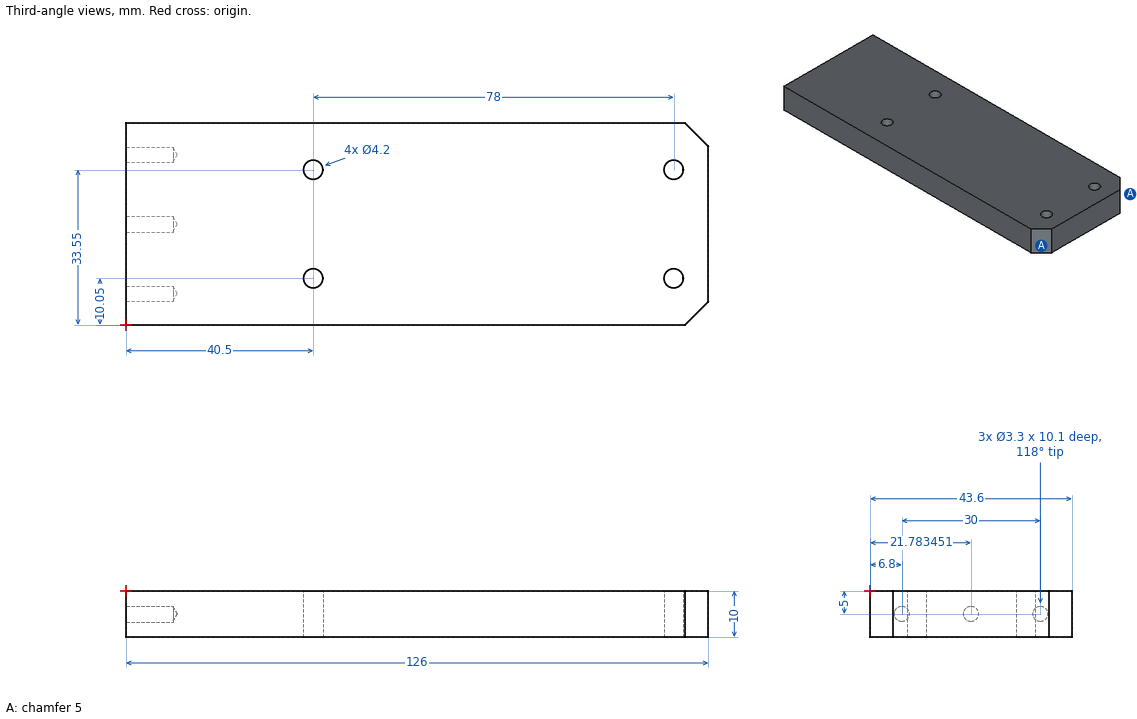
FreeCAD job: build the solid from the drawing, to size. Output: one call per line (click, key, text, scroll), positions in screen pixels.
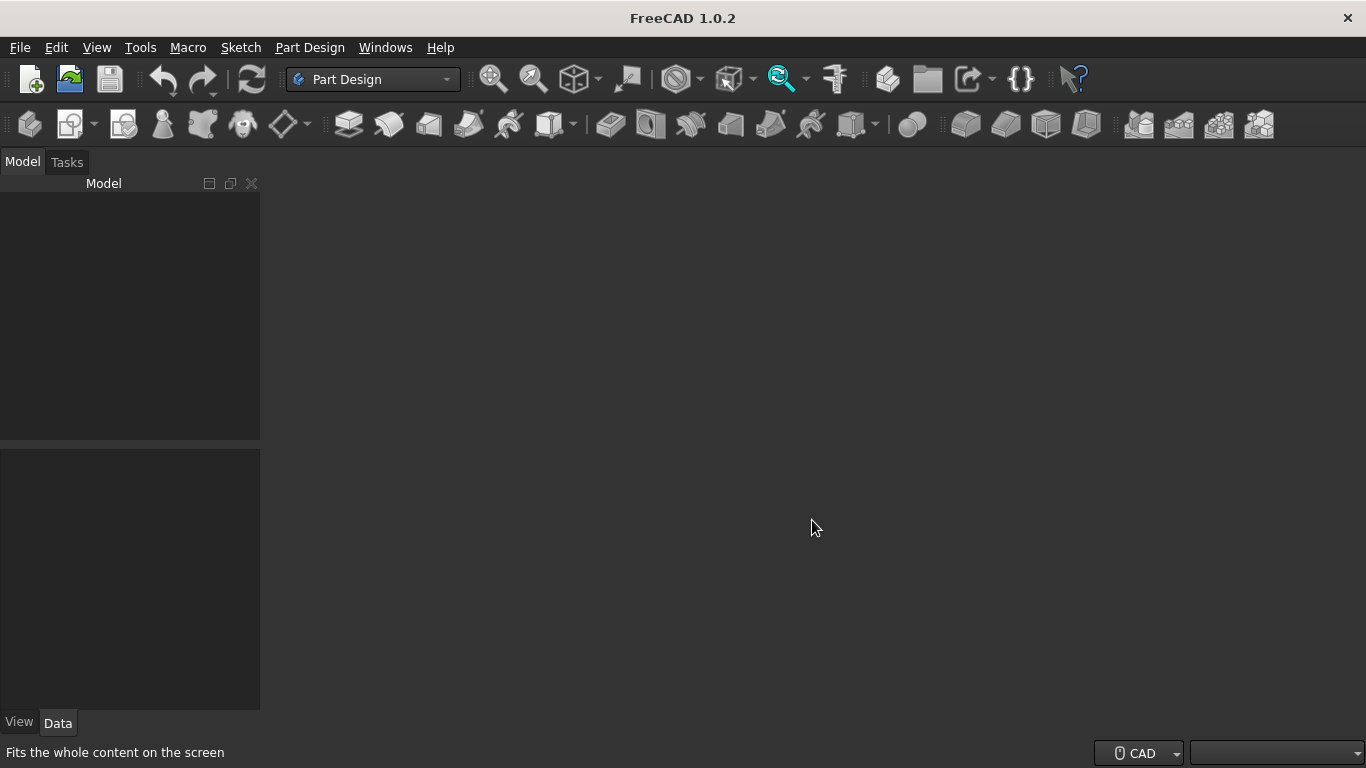
click(30, 80)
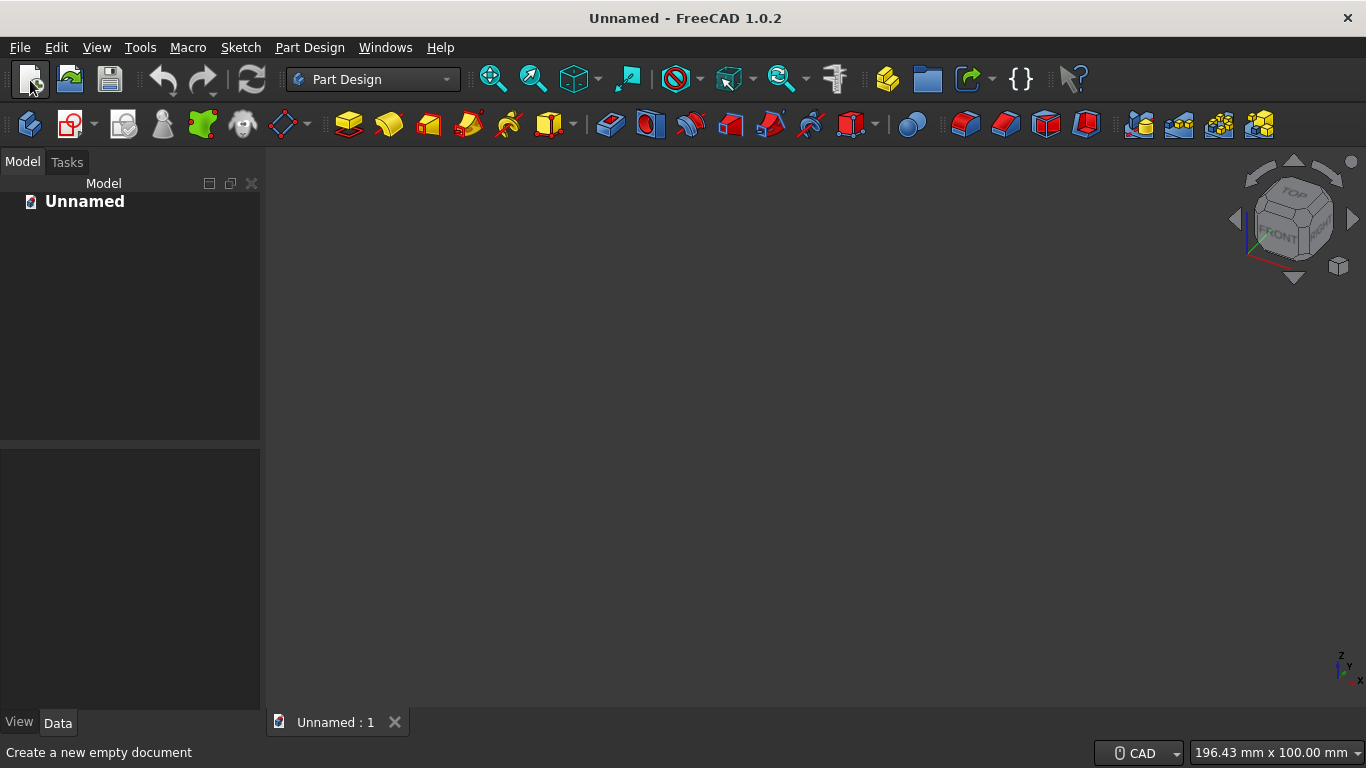
click(70, 124)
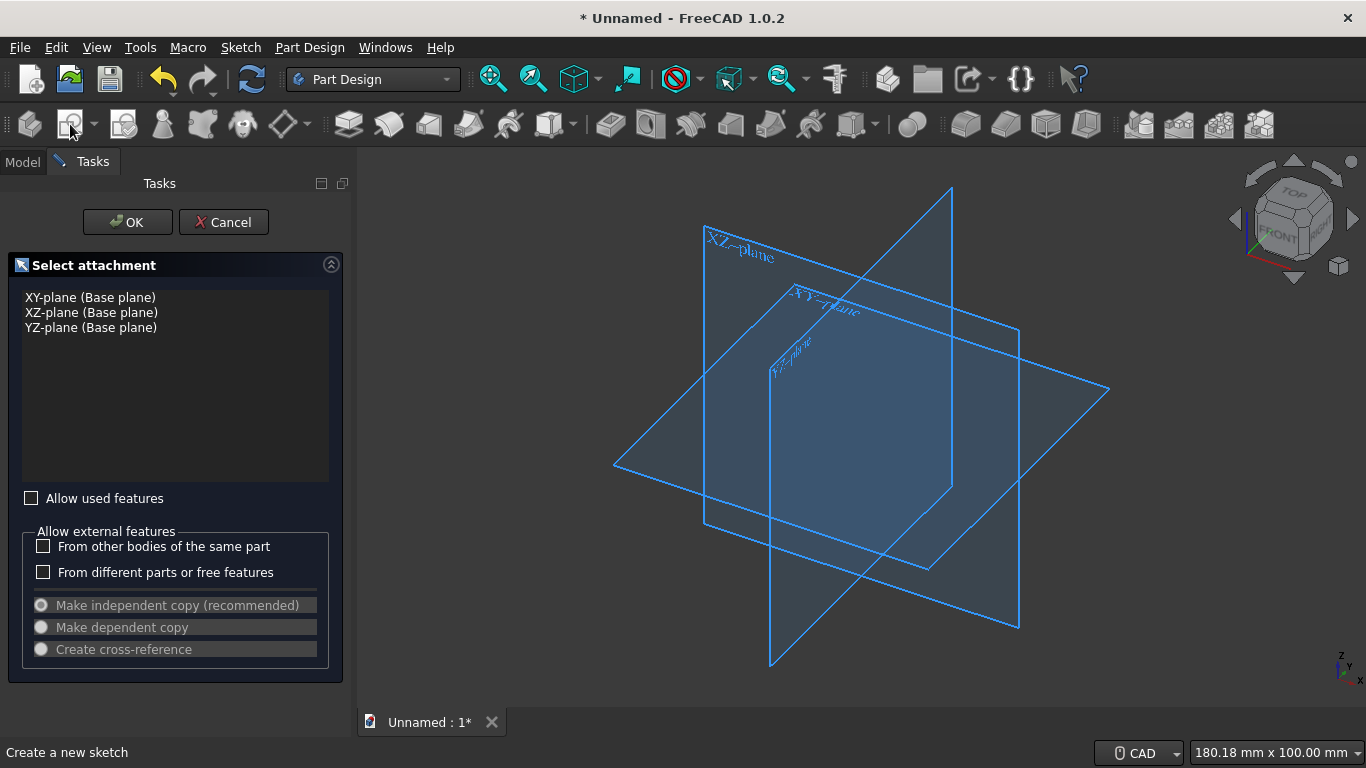
click(82, 312)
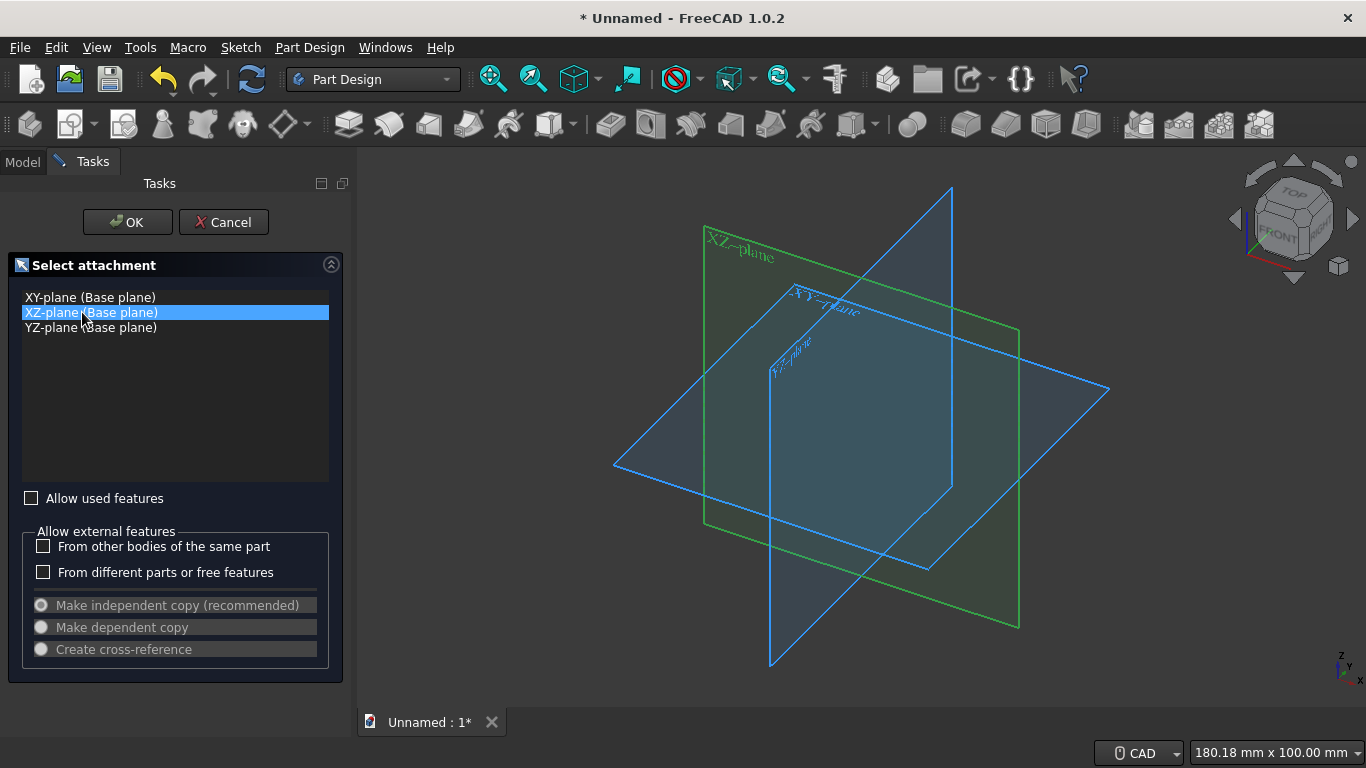
click(128, 222)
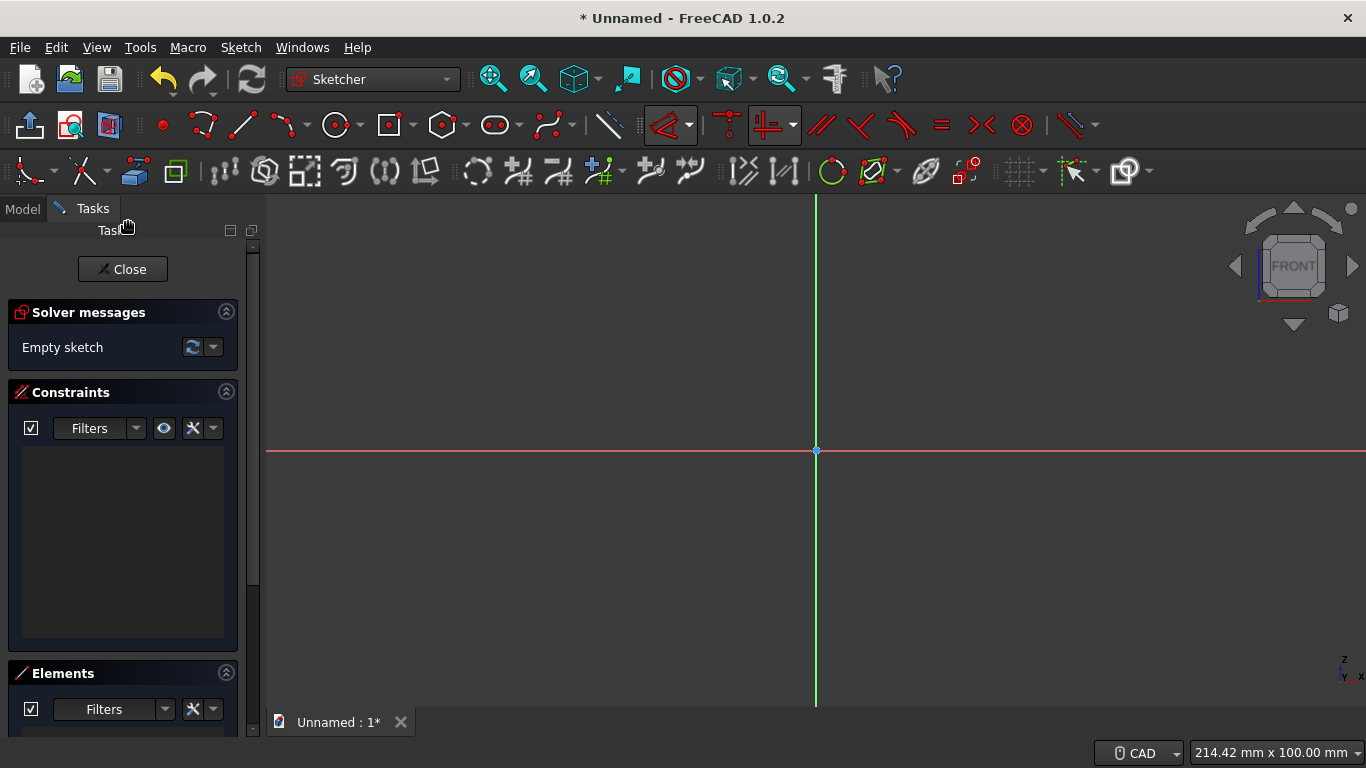
scroll(294, 398, down, 2)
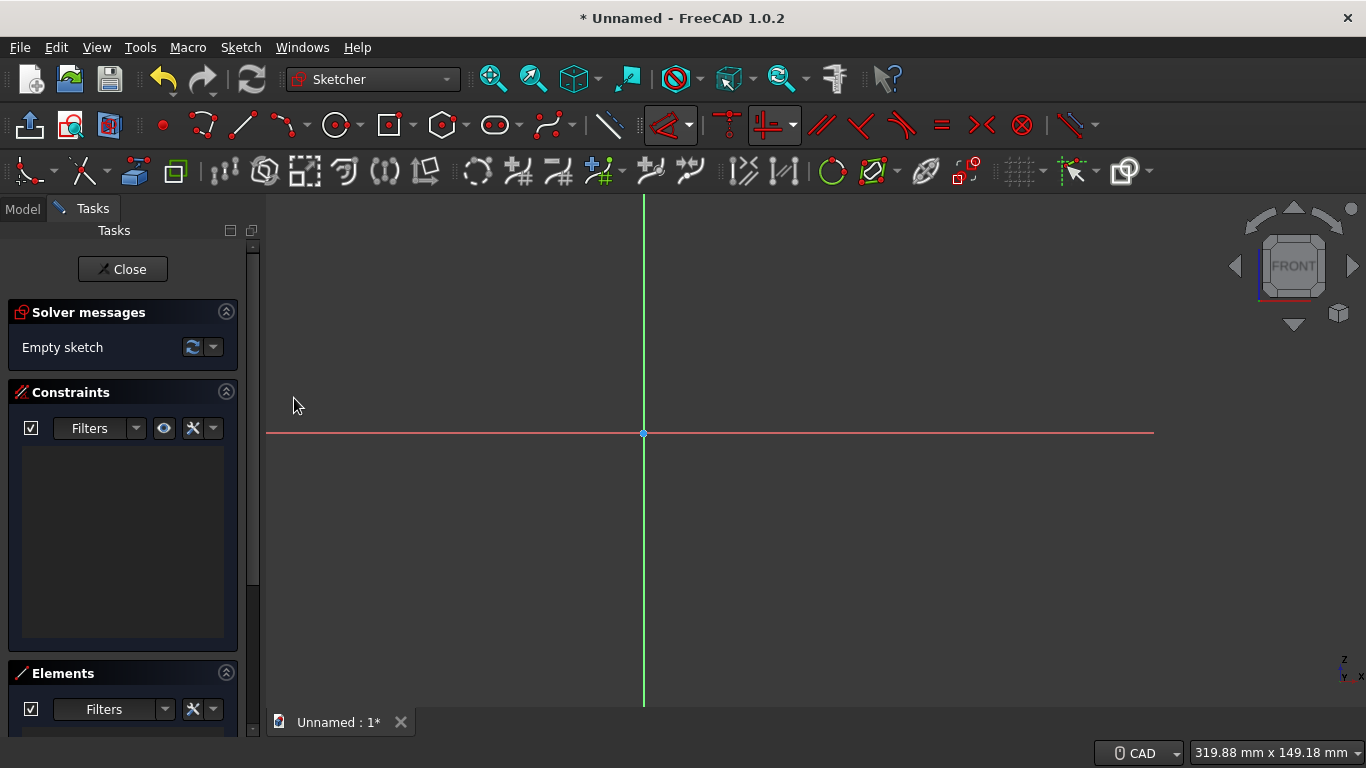
scroll(1090, 451, up, 2)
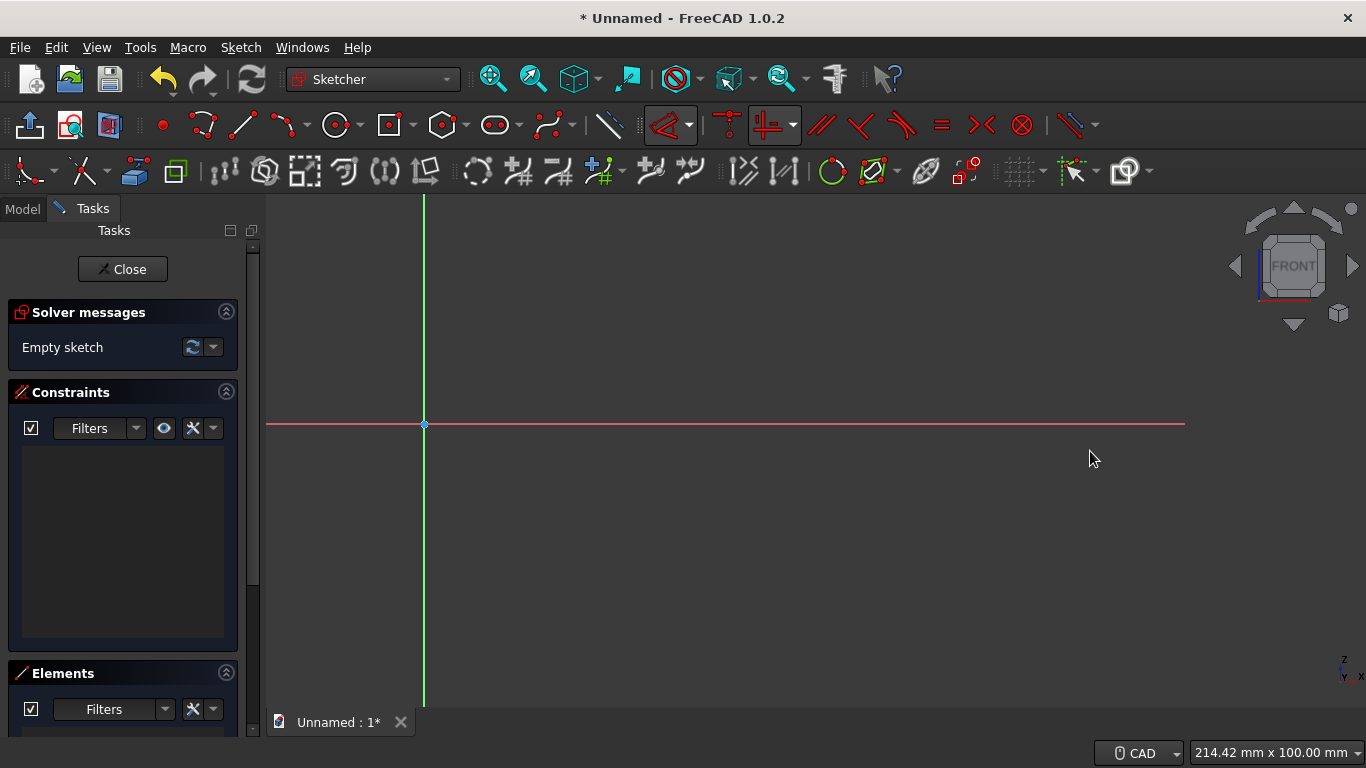
key(g)
key(r)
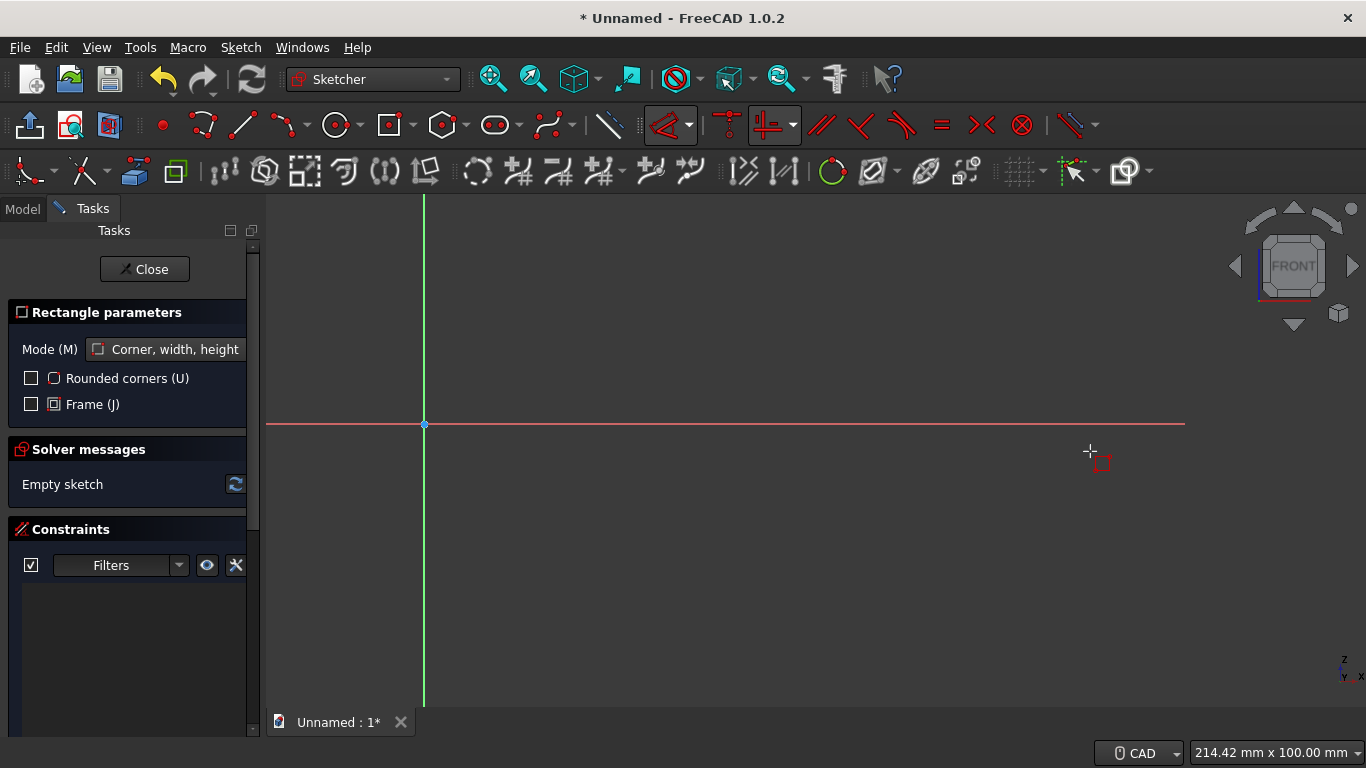
click(424, 424)
move(1071, 476)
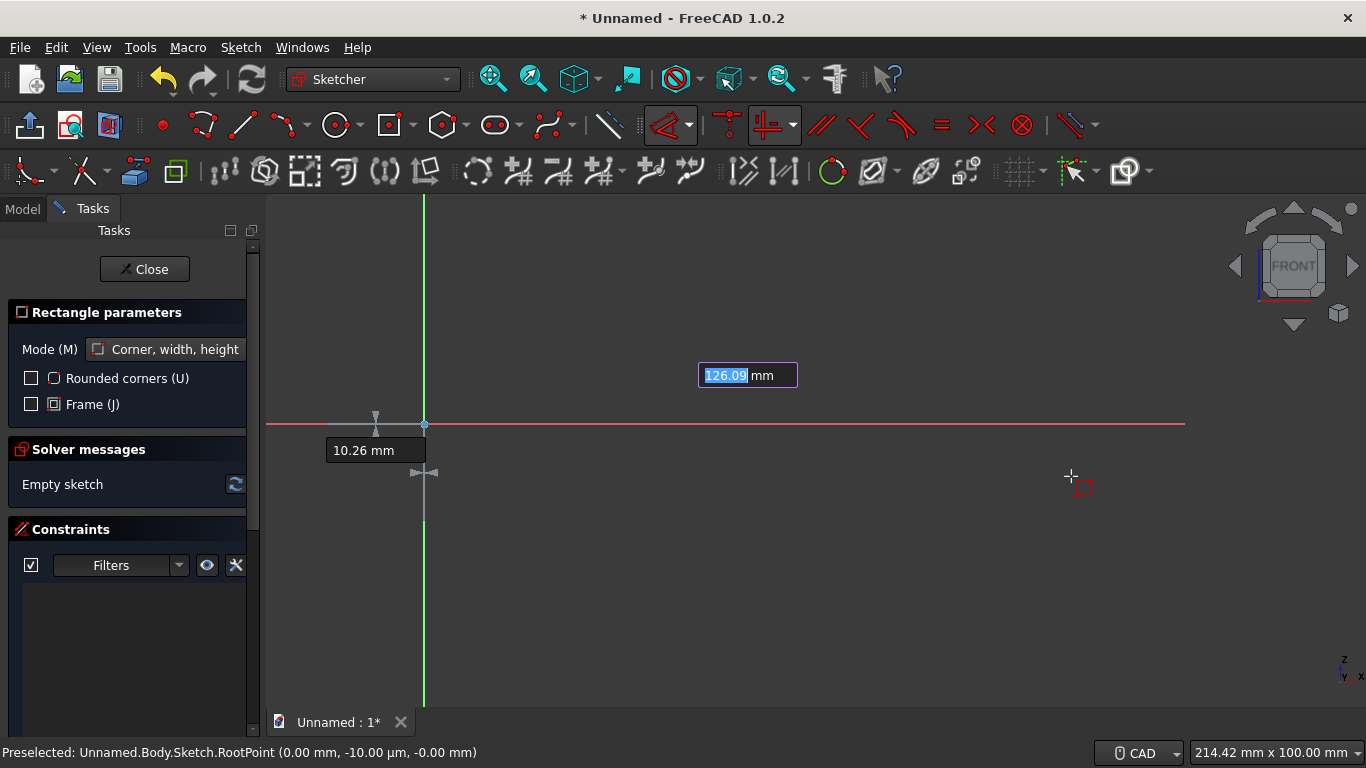
text(126)
key(Tab)
text(10)
key(Return)
key(Escape)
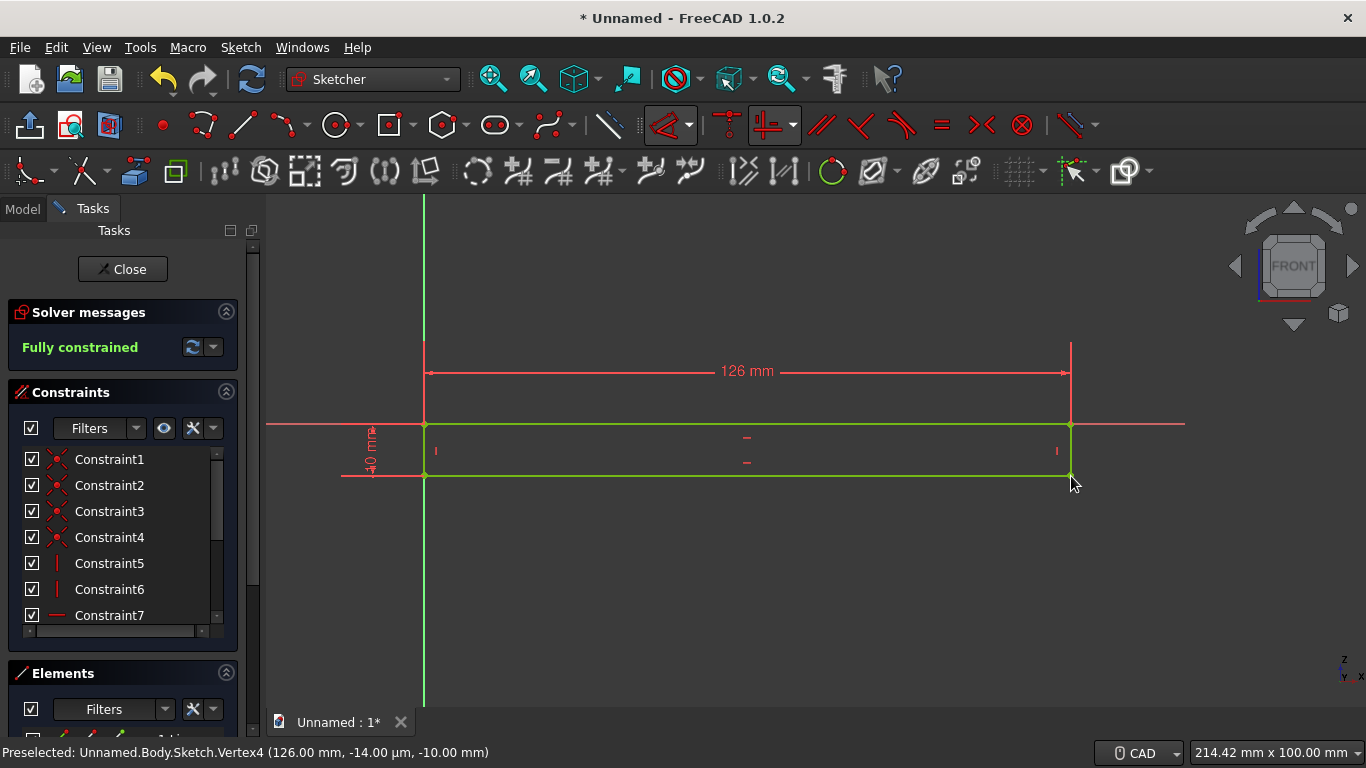
click(123, 269)